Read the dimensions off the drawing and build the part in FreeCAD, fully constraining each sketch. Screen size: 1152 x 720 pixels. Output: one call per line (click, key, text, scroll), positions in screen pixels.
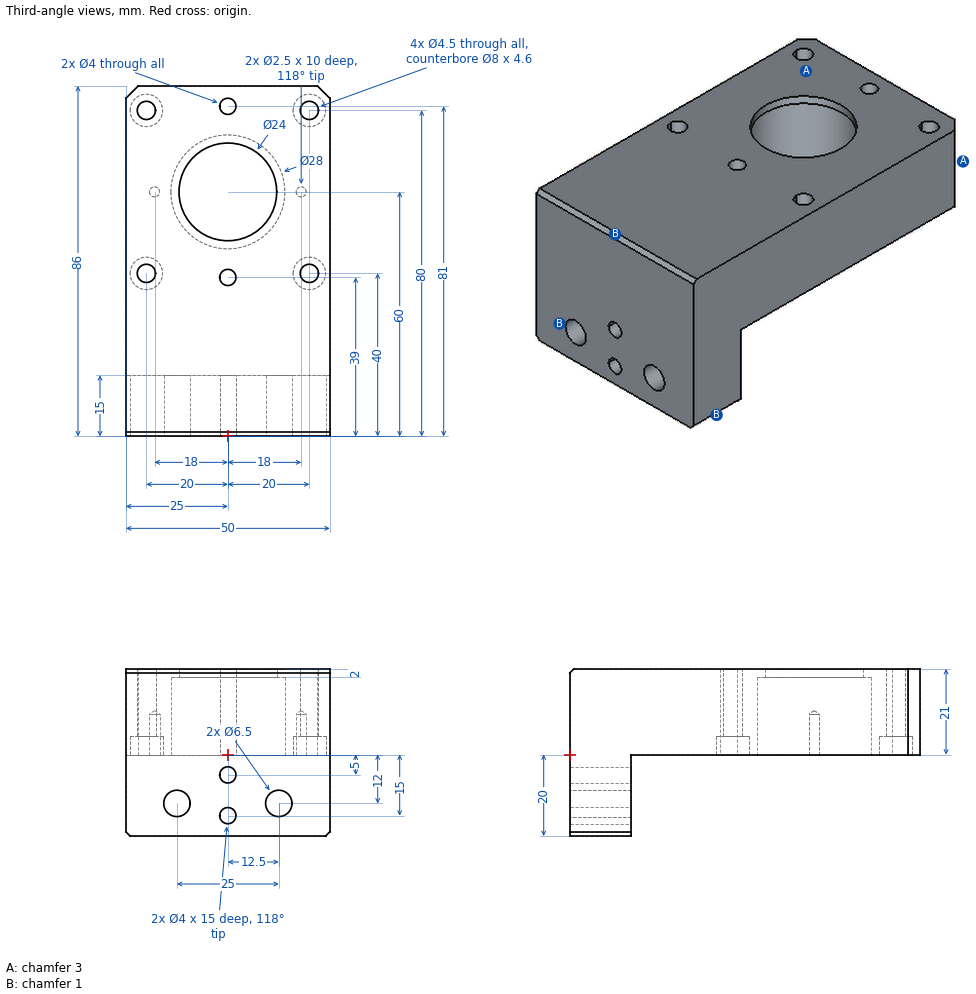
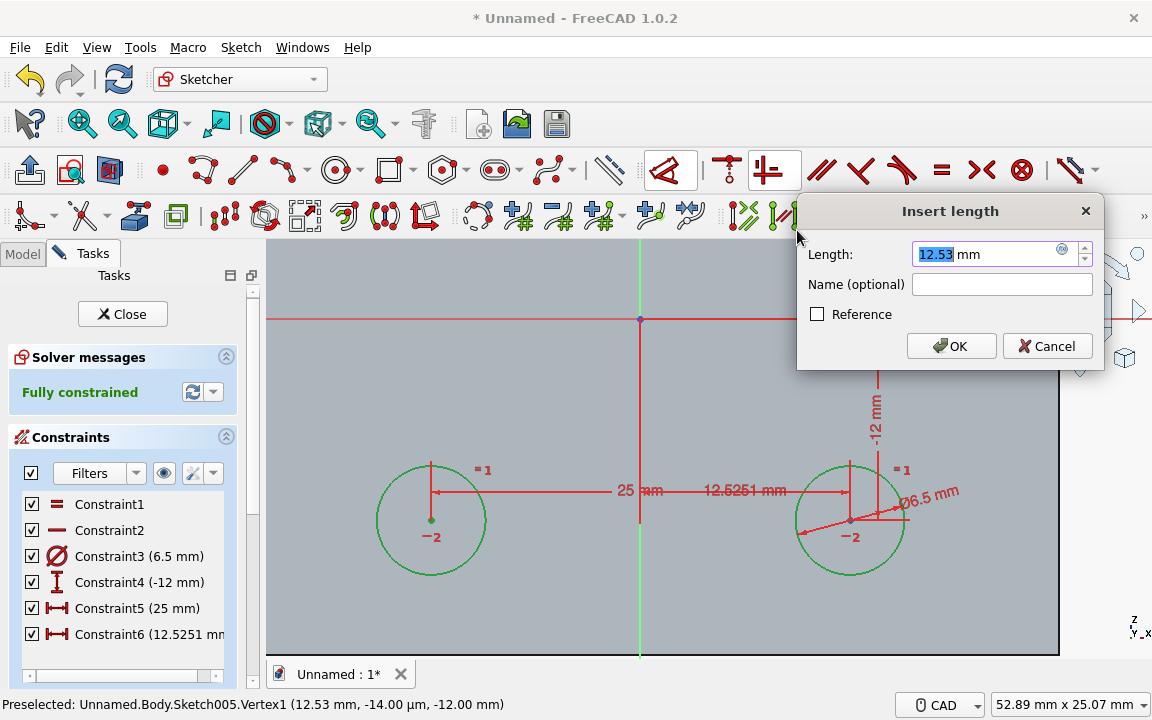
text(12.5)
key(Return)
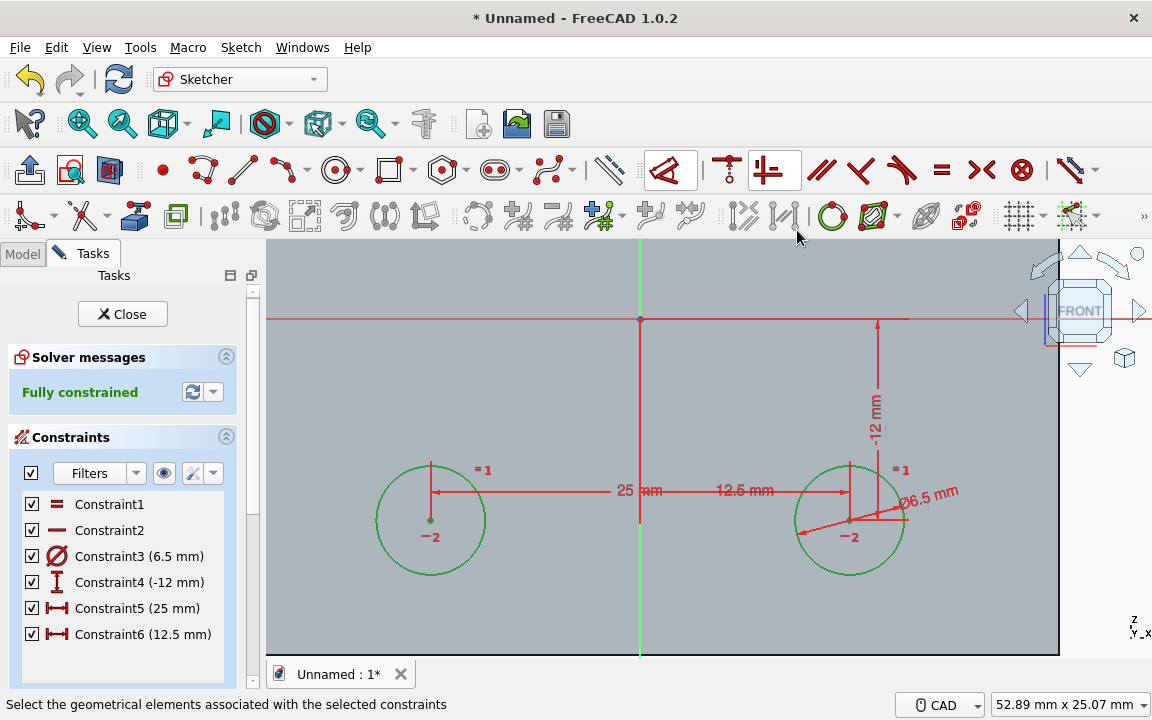
click(123, 314)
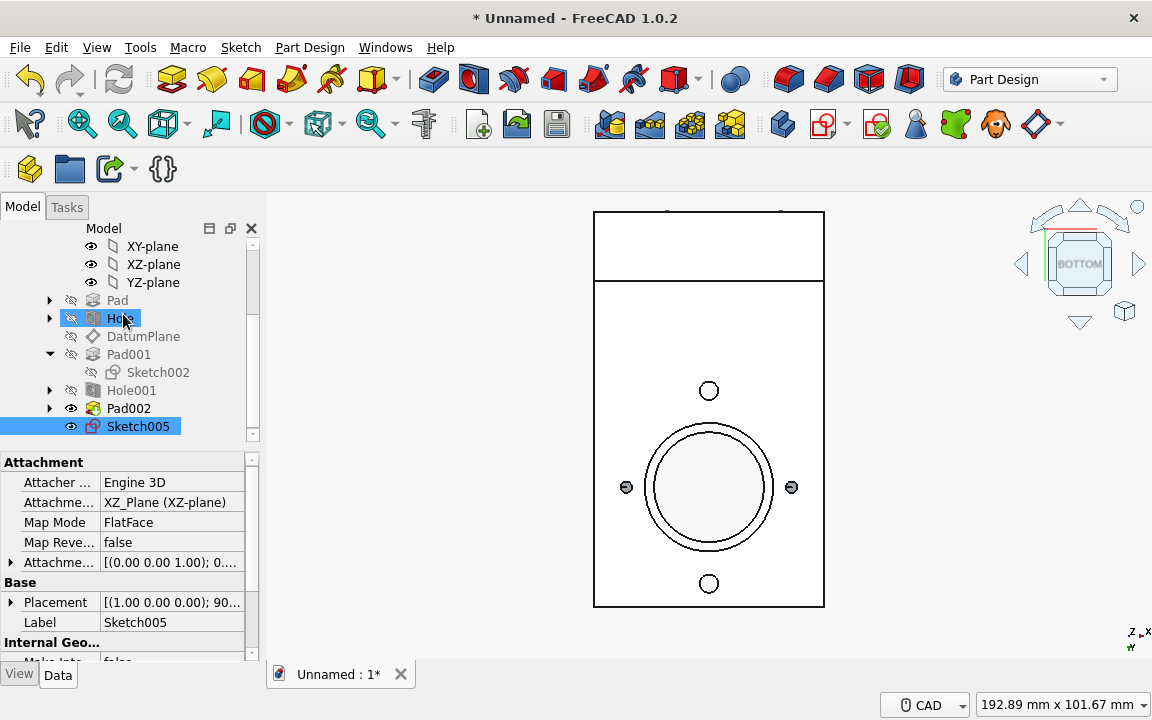
click(434, 80)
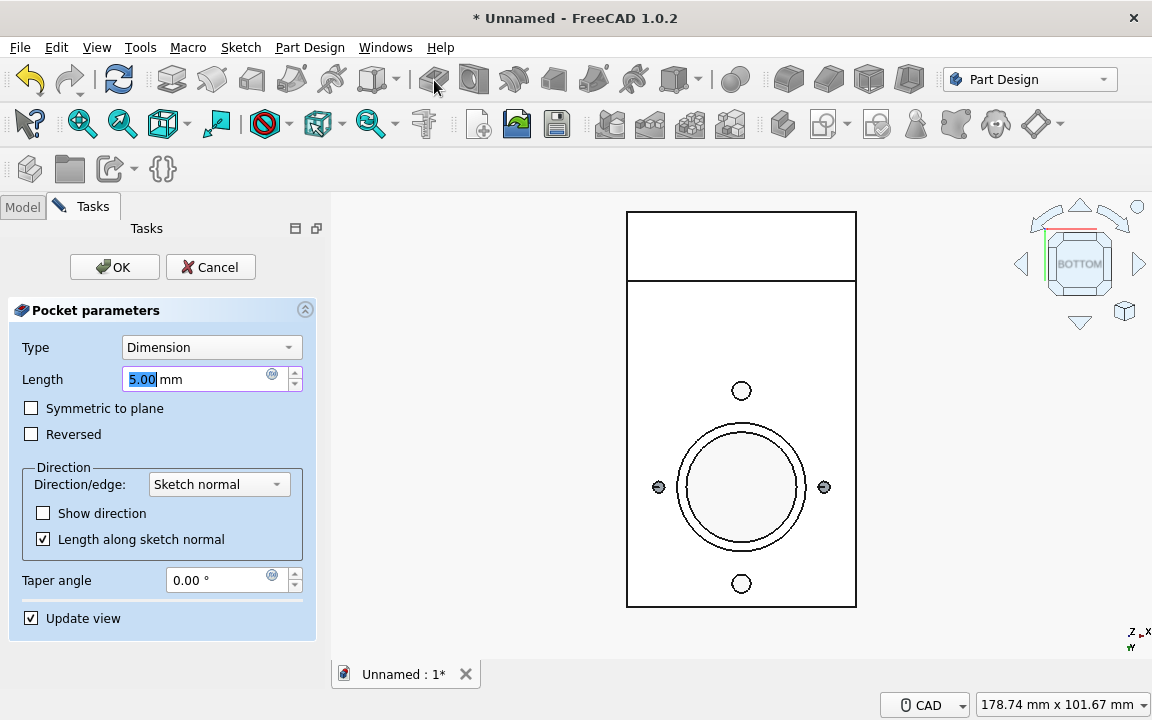
click(212, 348)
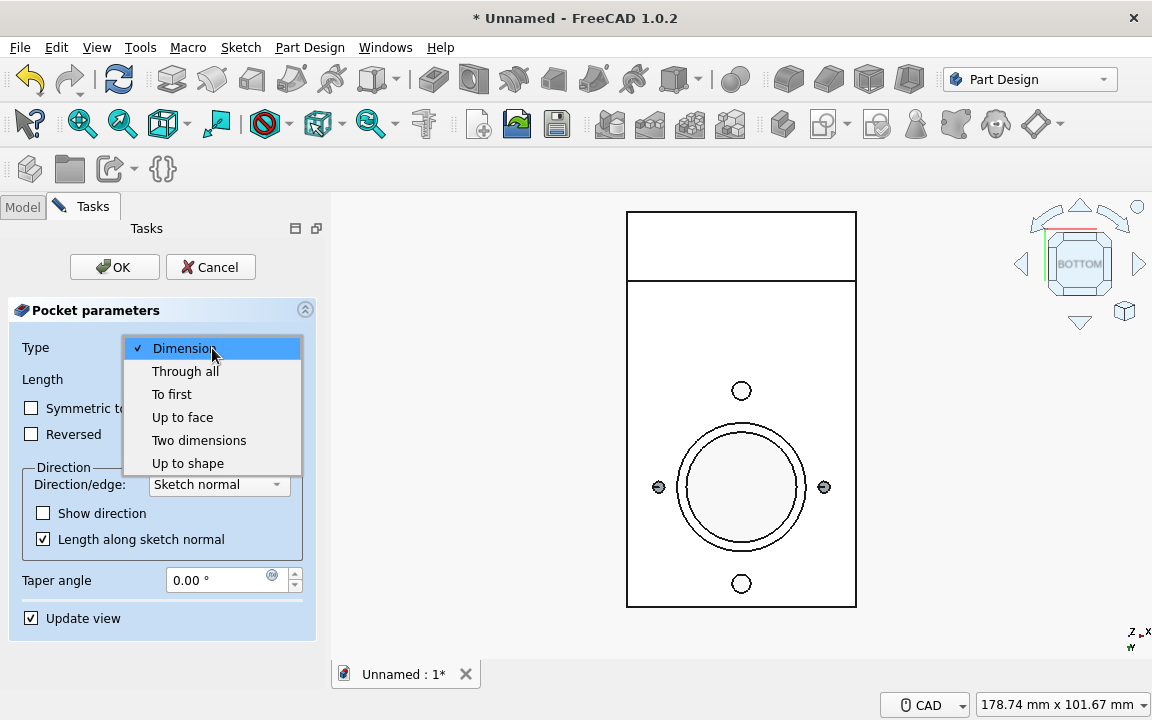
click(212, 372)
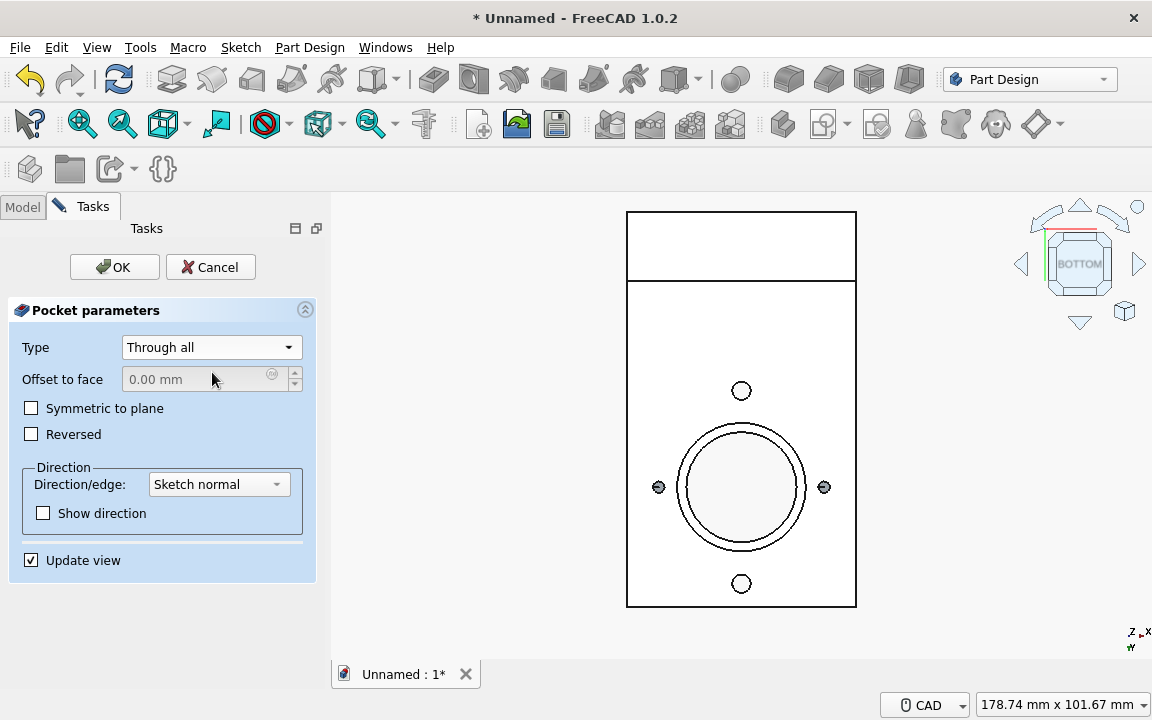
click(115, 267)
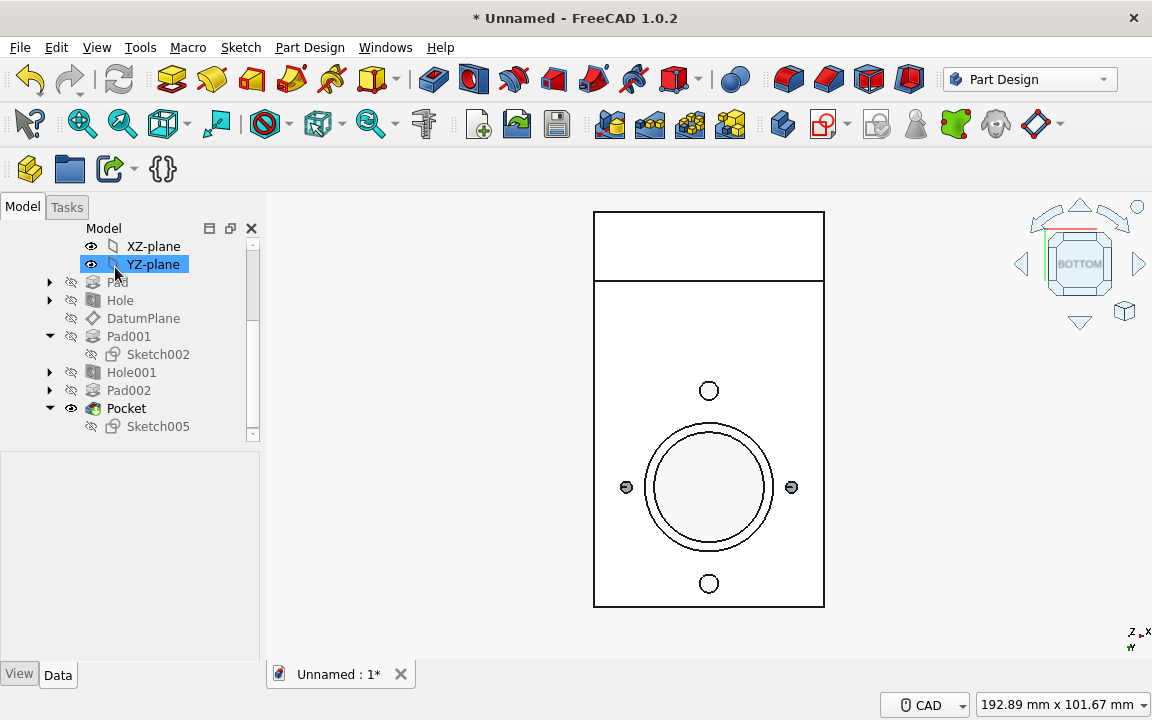
key(0)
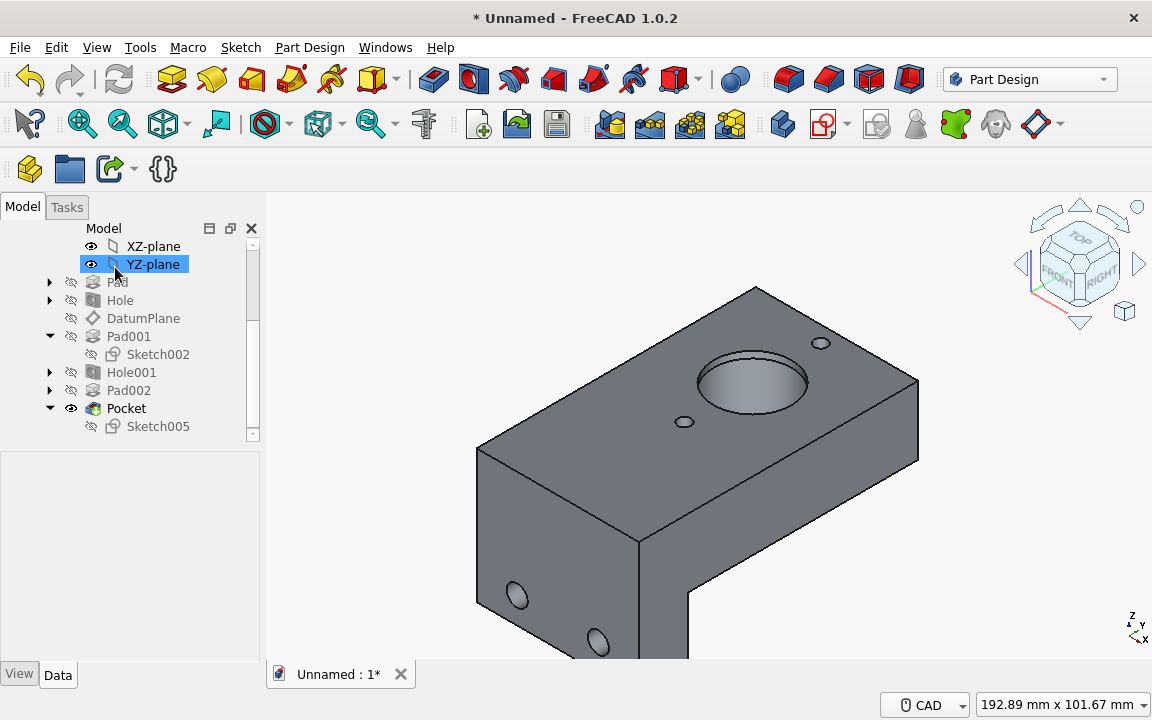
key(v)
key(f)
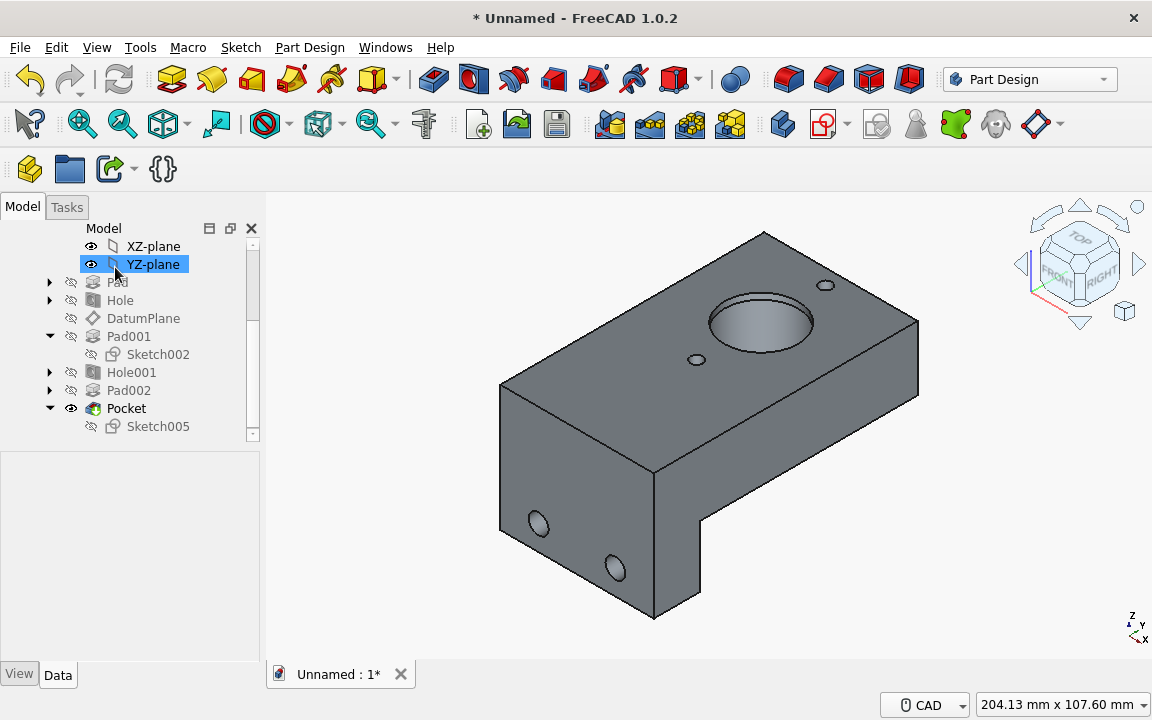
click(599, 493)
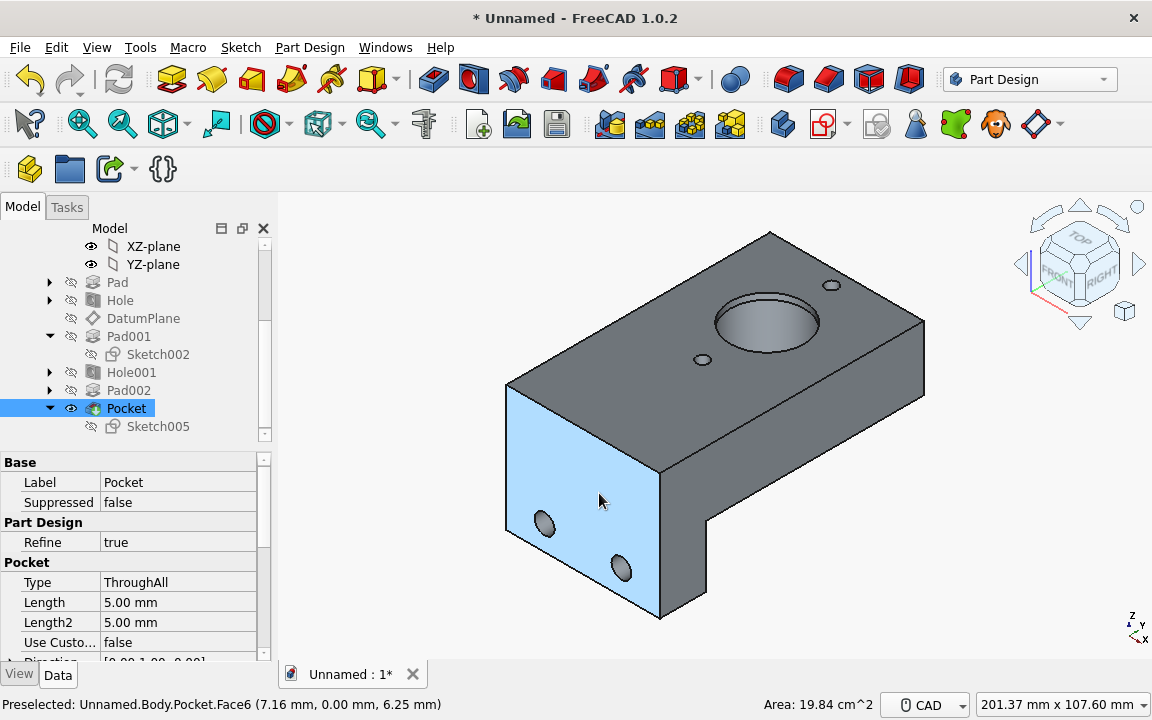
click(824, 124)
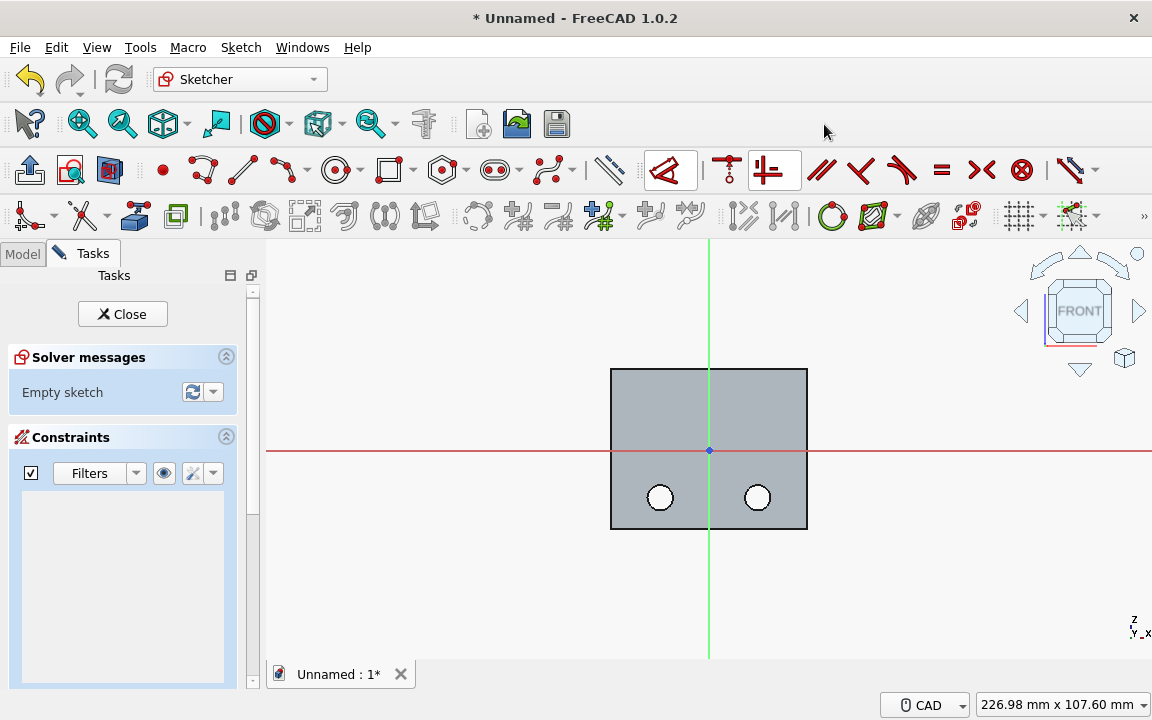
scroll(731, 496, up, 7)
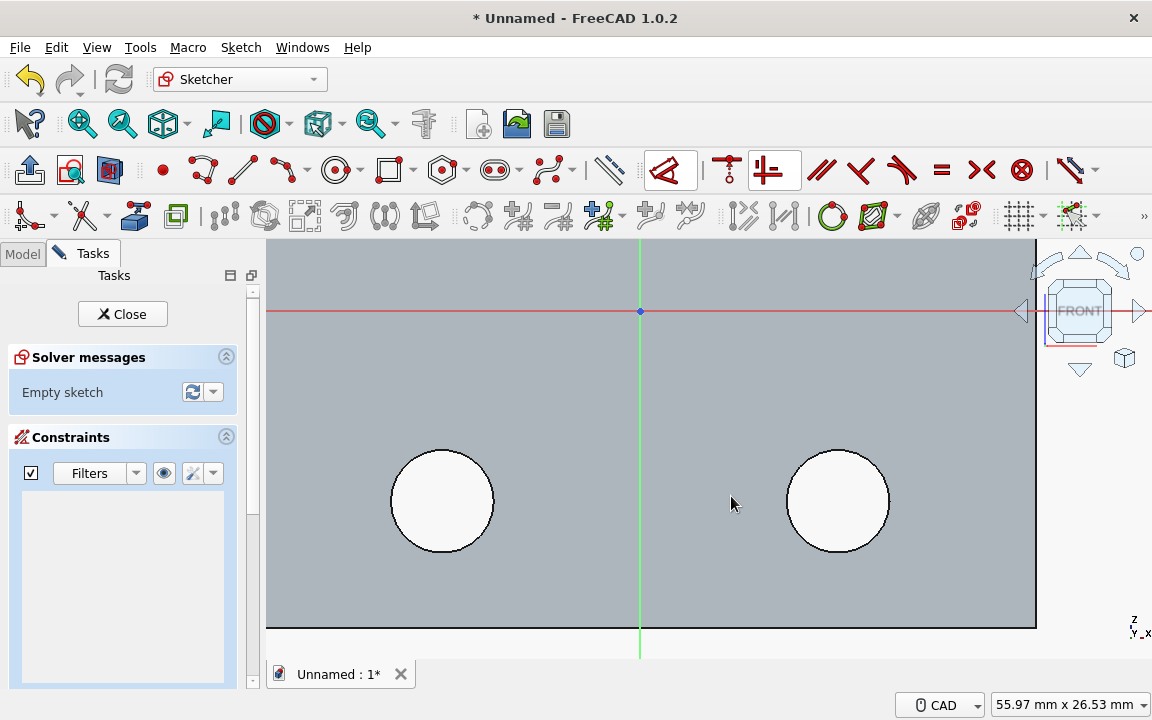
click(336, 170)